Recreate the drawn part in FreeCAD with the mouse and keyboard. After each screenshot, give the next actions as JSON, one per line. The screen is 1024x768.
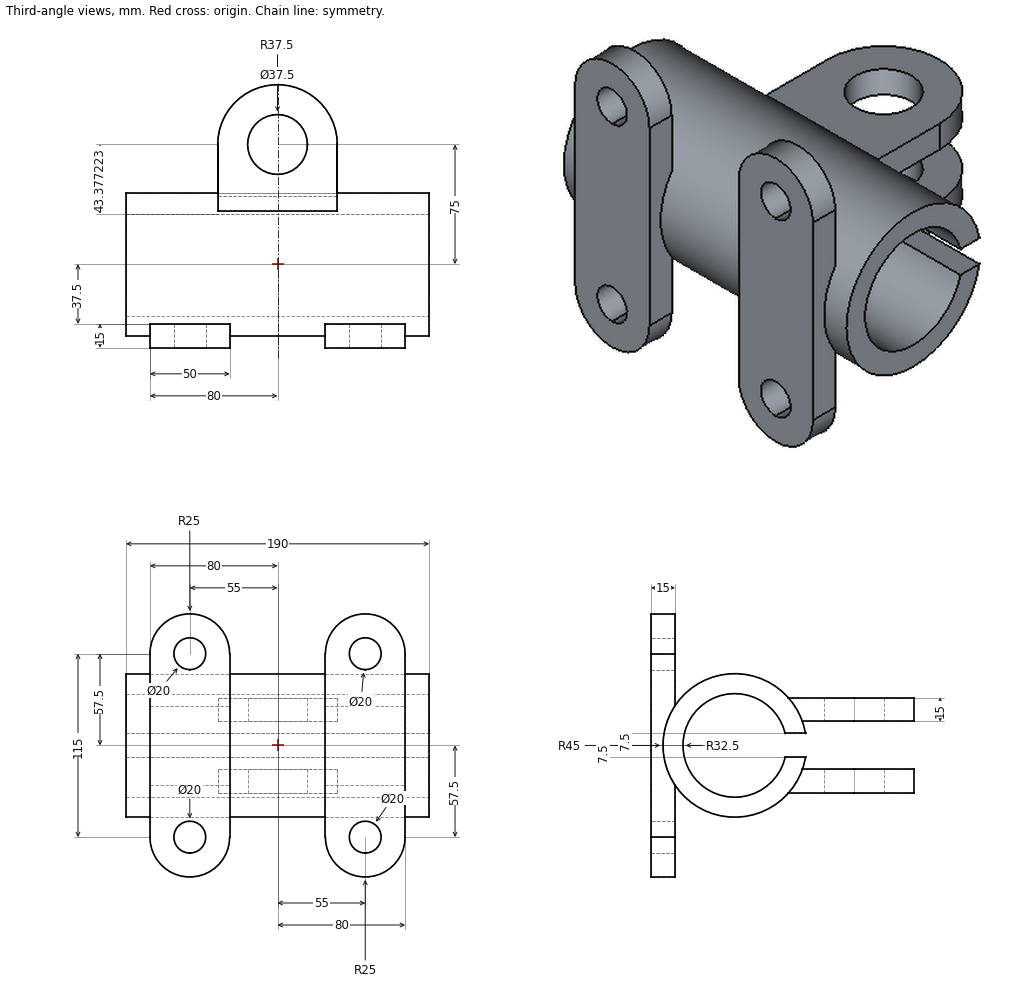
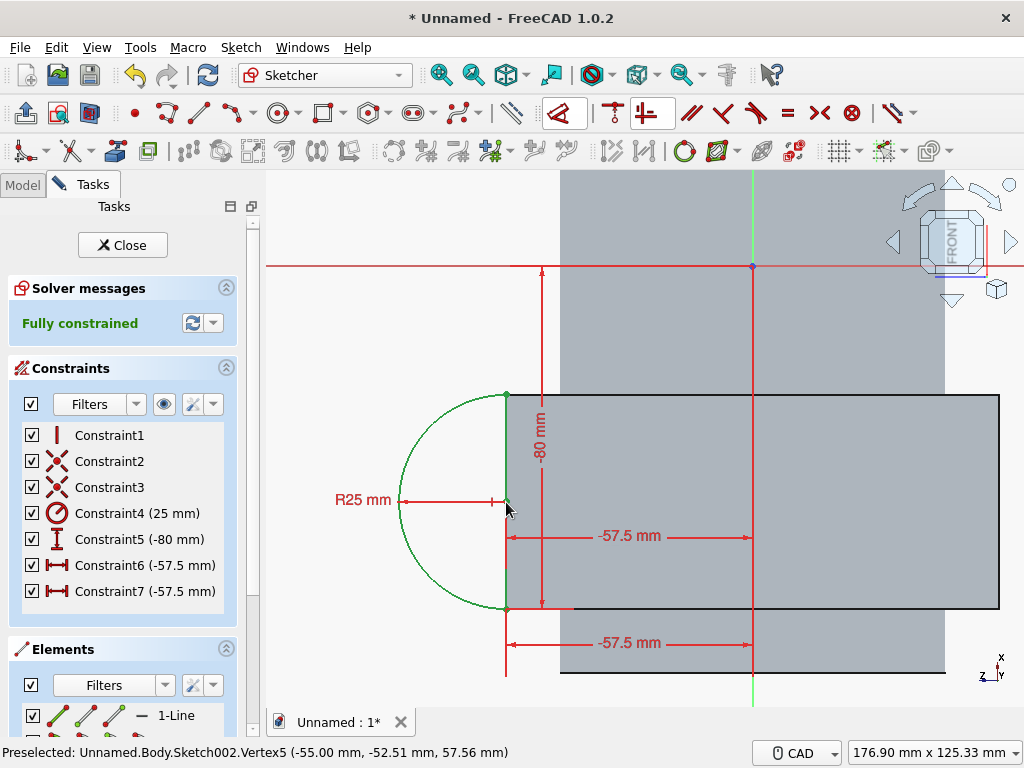
{"action": "left_click", "coordinate": [123, 245]}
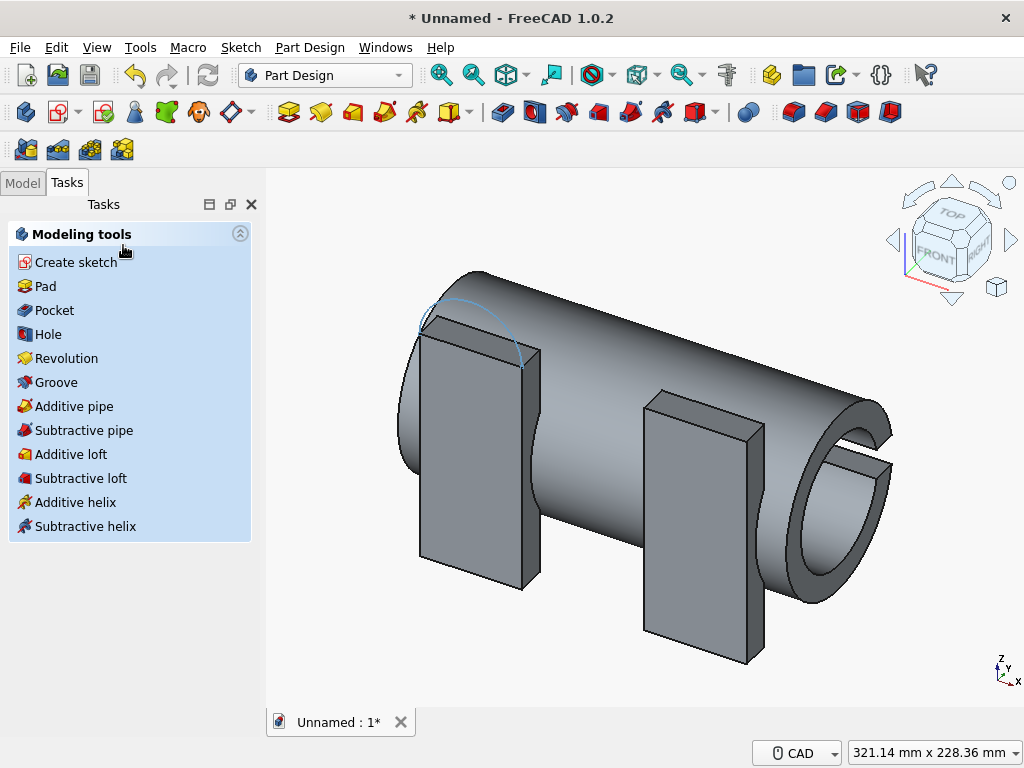
{"action": "left_click", "coordinate": [290, 112]}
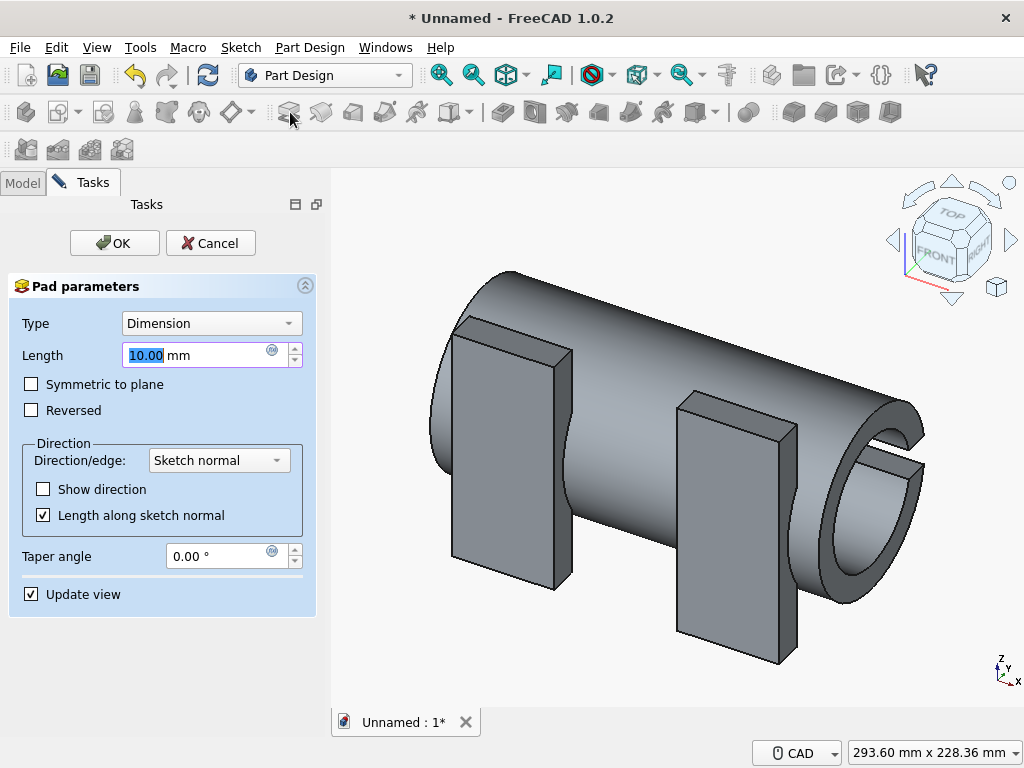
{"action": "type", "text": "15"}
{"action": "key", "text": "Tab"}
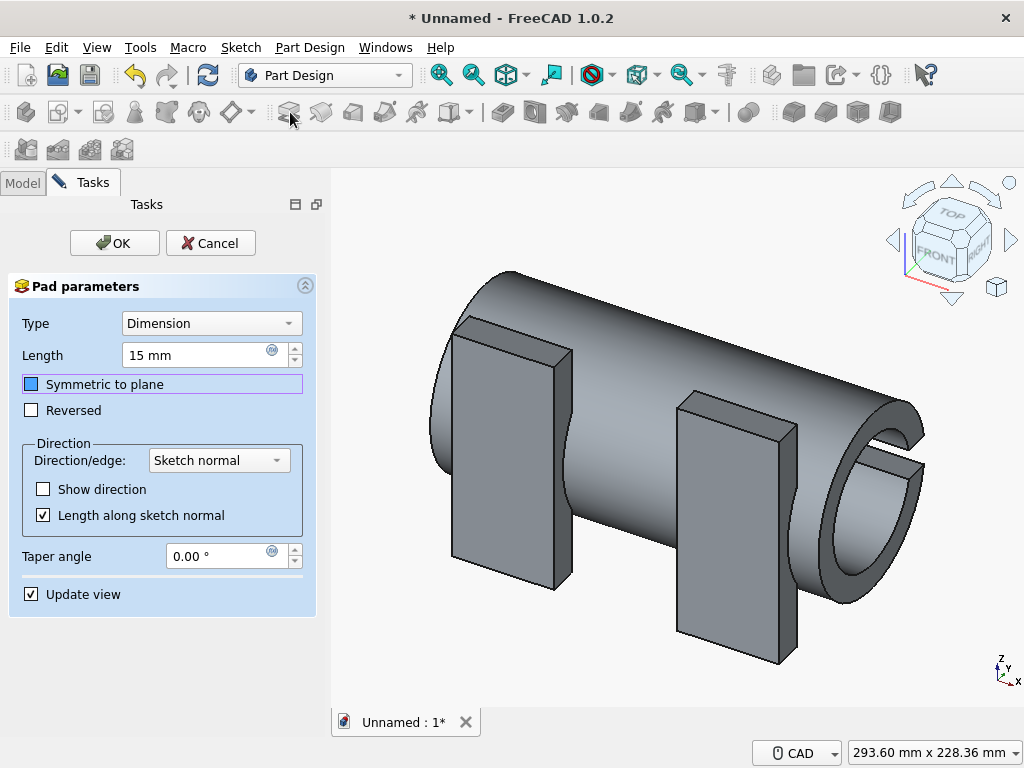
{"action": "left_click", "coordinate": [30, 410]}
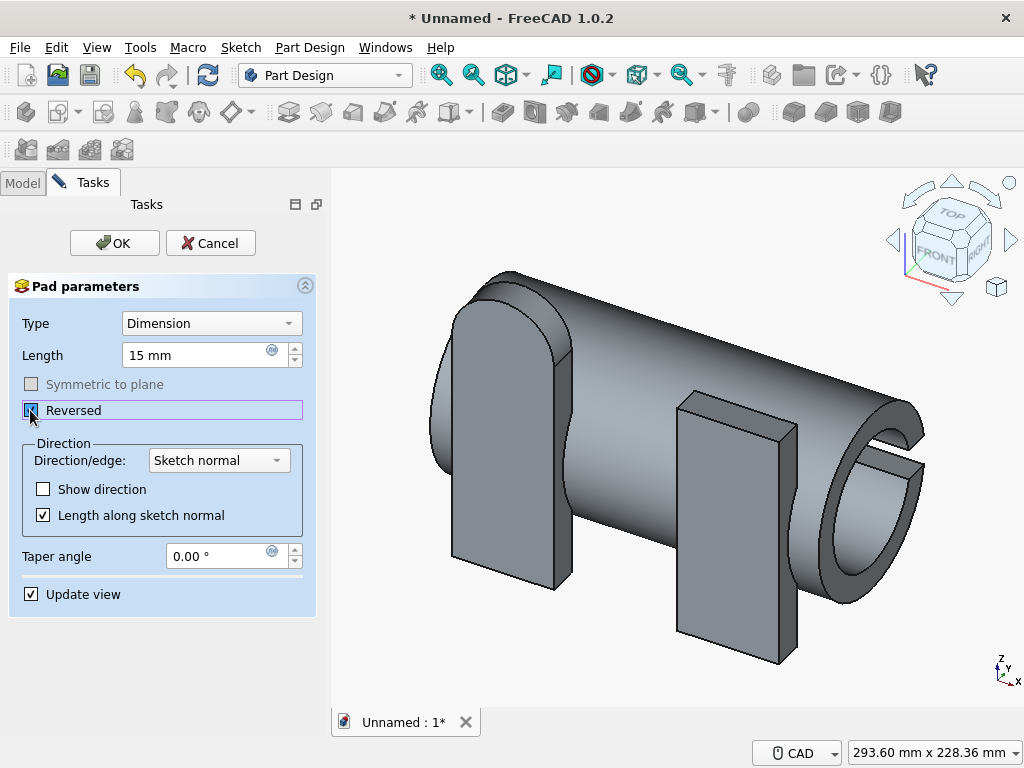
{"action": "left_click", "coordinate": [115, 243]}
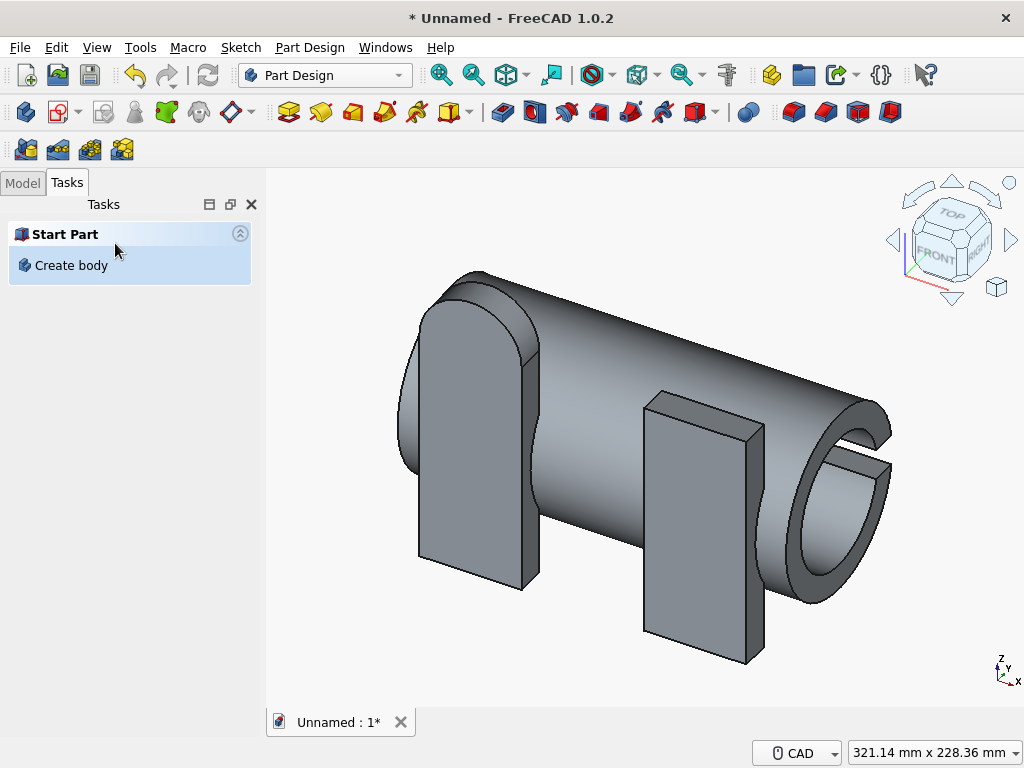
{"action": "left_click", "coordinate": [442, 76]}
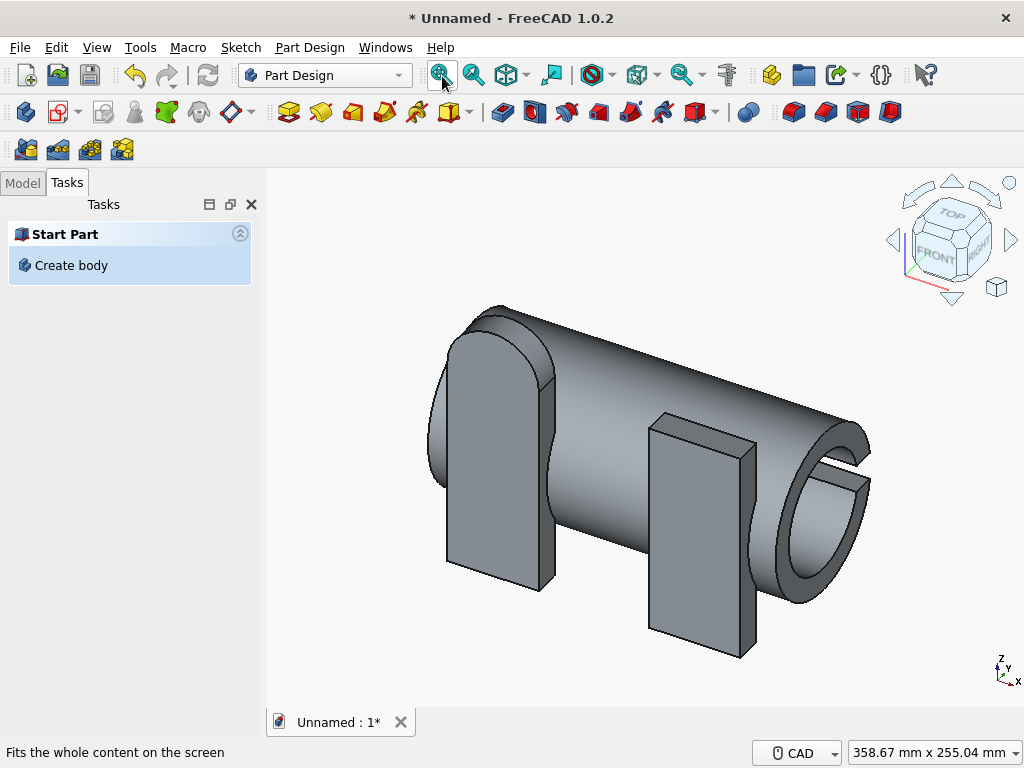
{"action": "left_click", "coordinate": [23, 182]}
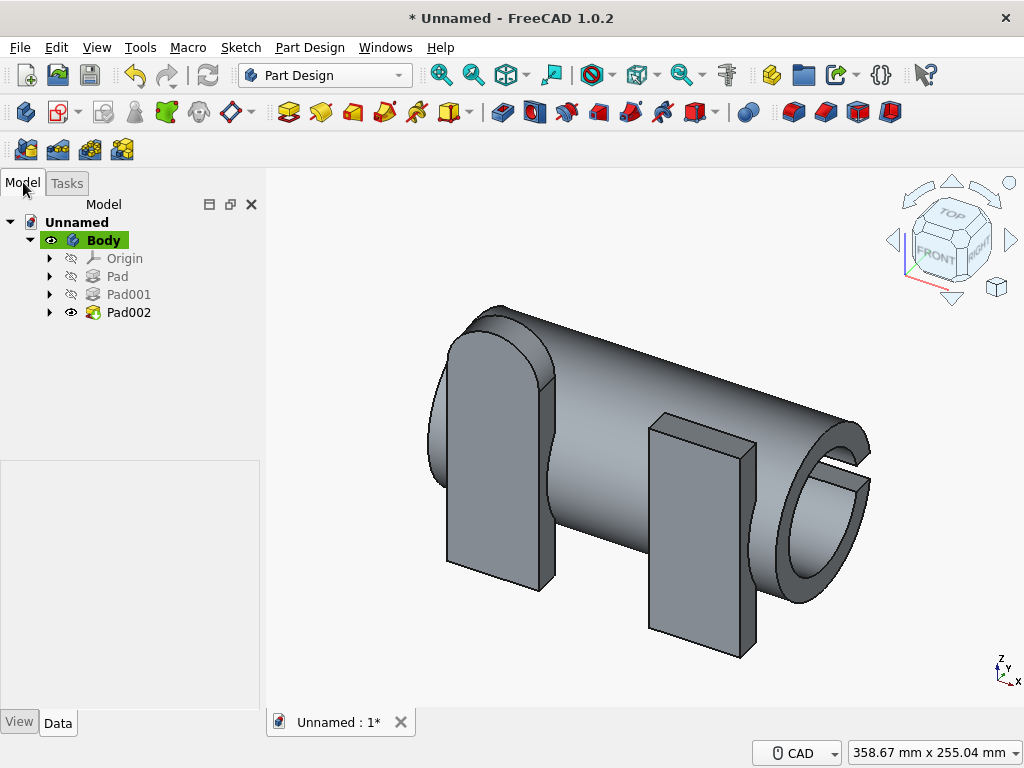
{"action": "left_click", "coordinate": [116, 312]}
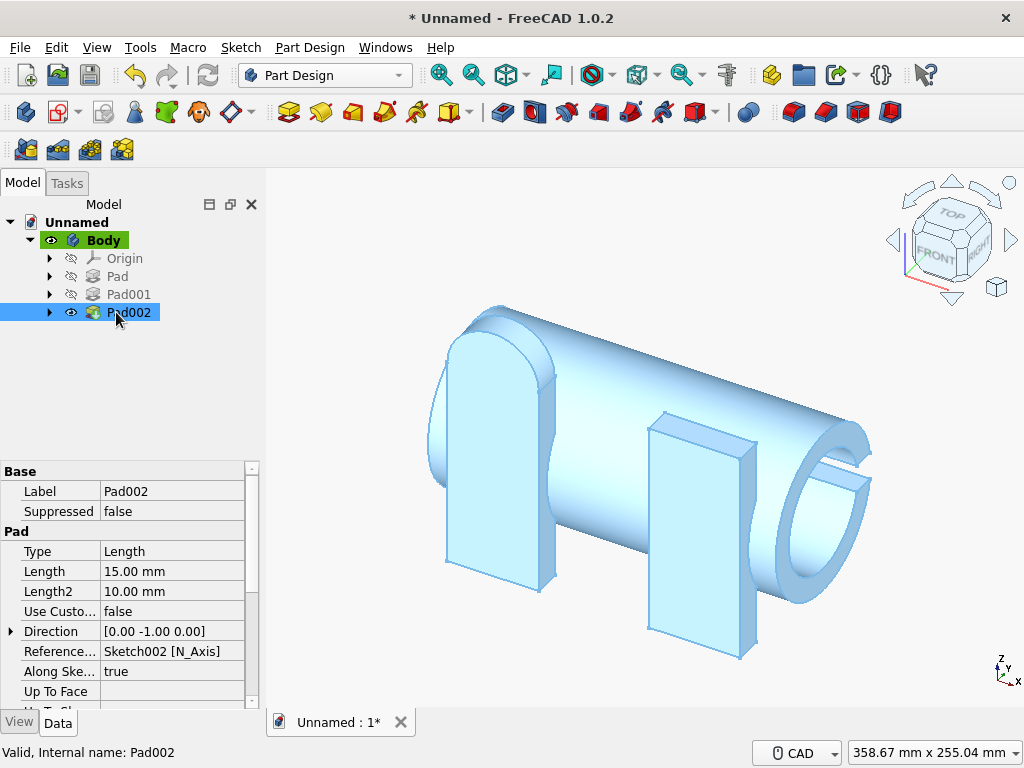
{"action": "left_click", "coordinate": [26, 150]}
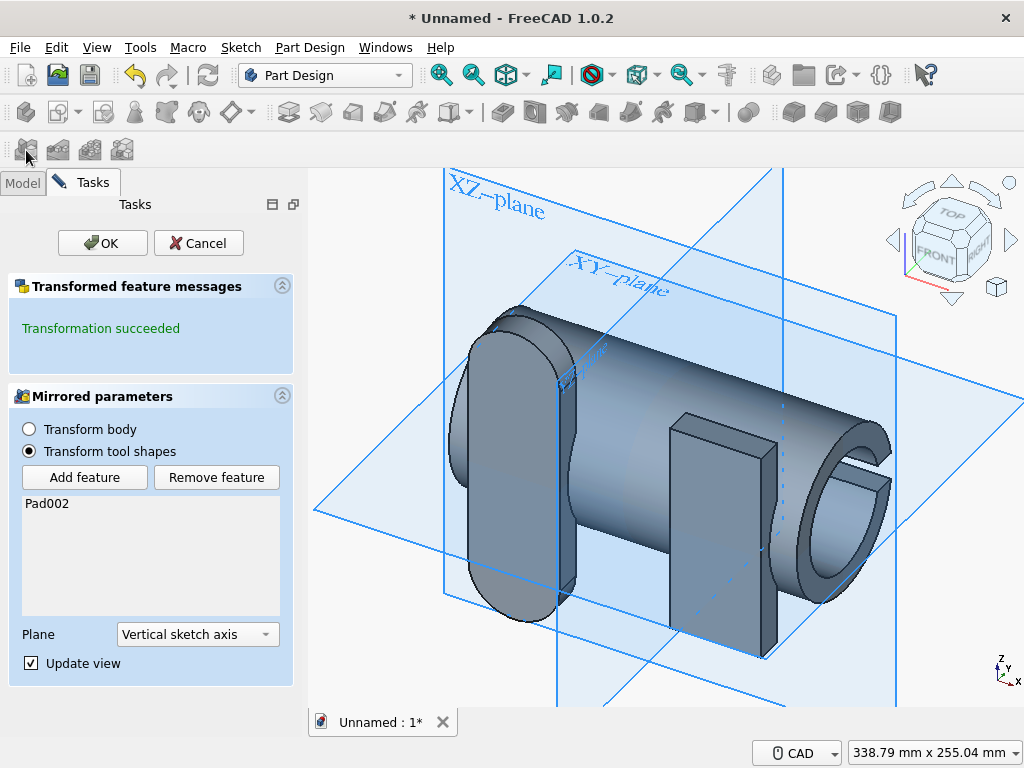
{"action": "left_click", "coordinate": [198, 634]}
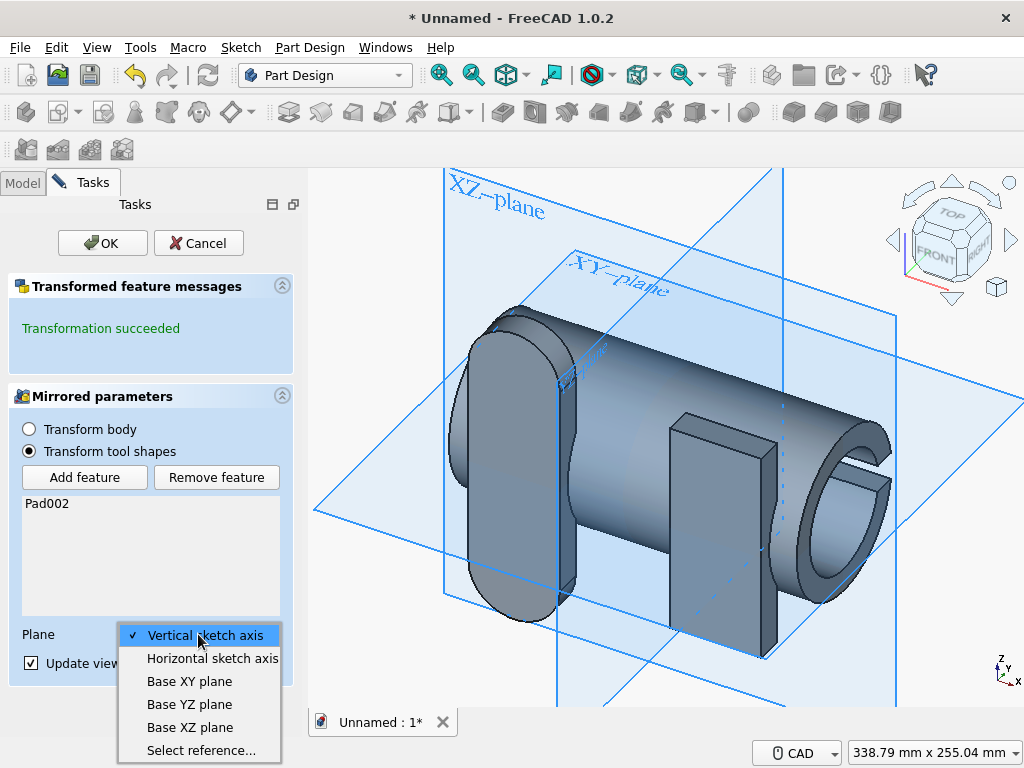
{"action": "left_click", "coordinate": [198, 682]}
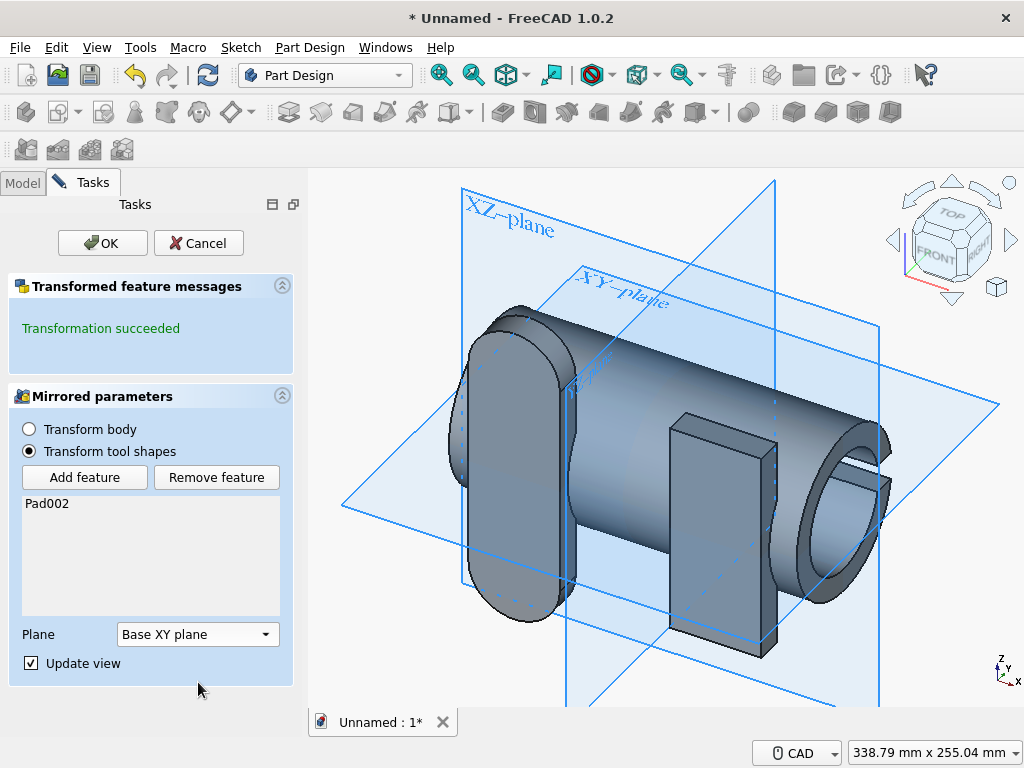
{"action": "left_click", "coordinate": [103, 243]}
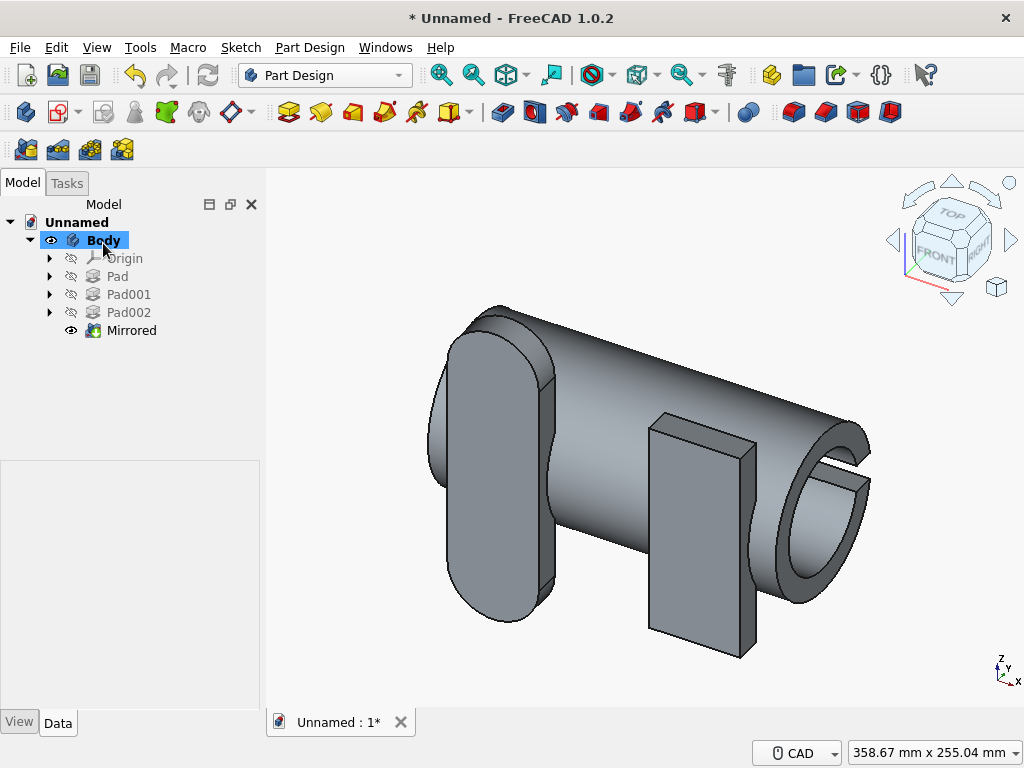
{"action": "left_click", "coordinate": [442, 76]}